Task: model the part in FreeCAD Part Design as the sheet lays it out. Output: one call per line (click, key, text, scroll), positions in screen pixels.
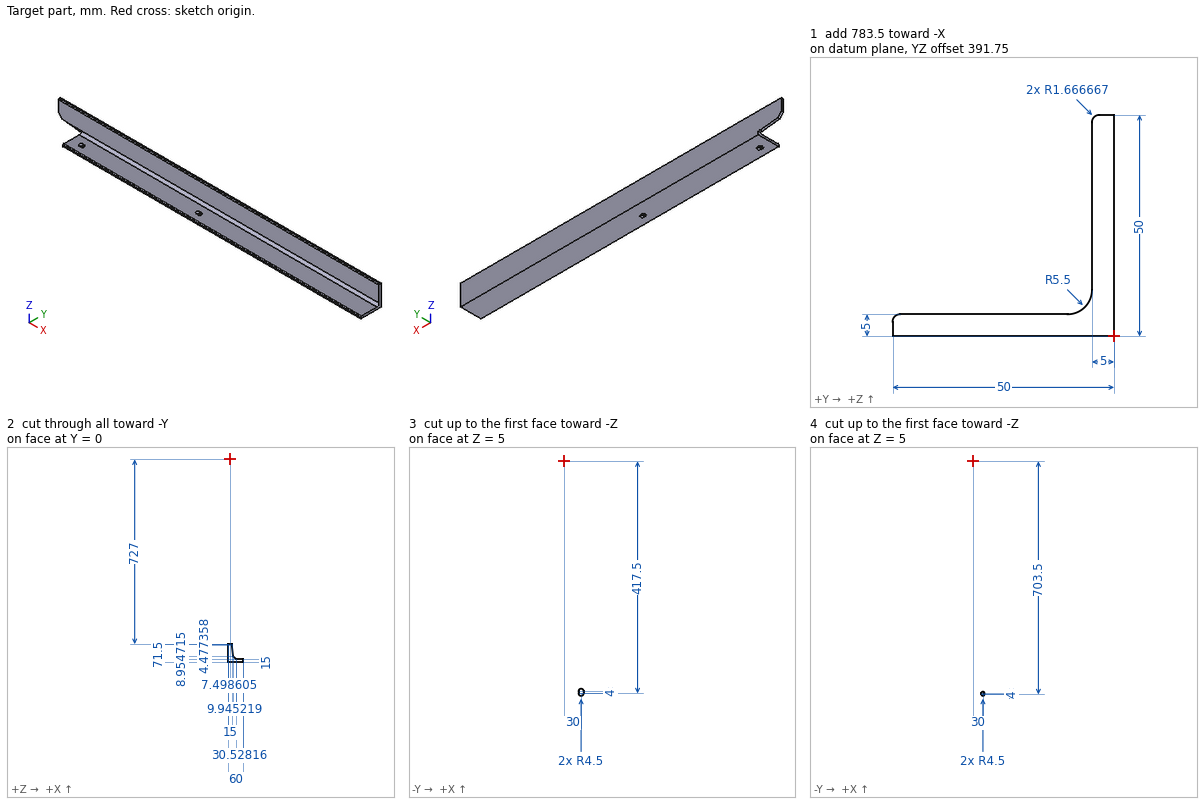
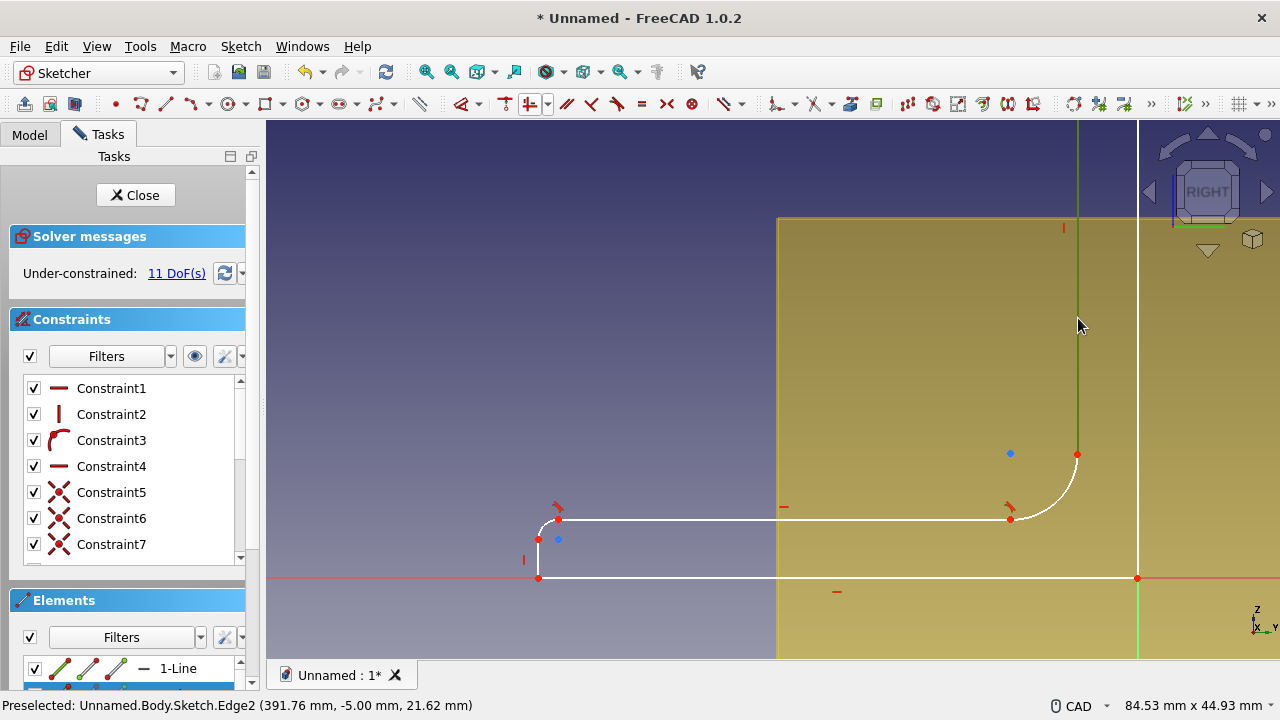
click(1041, 513)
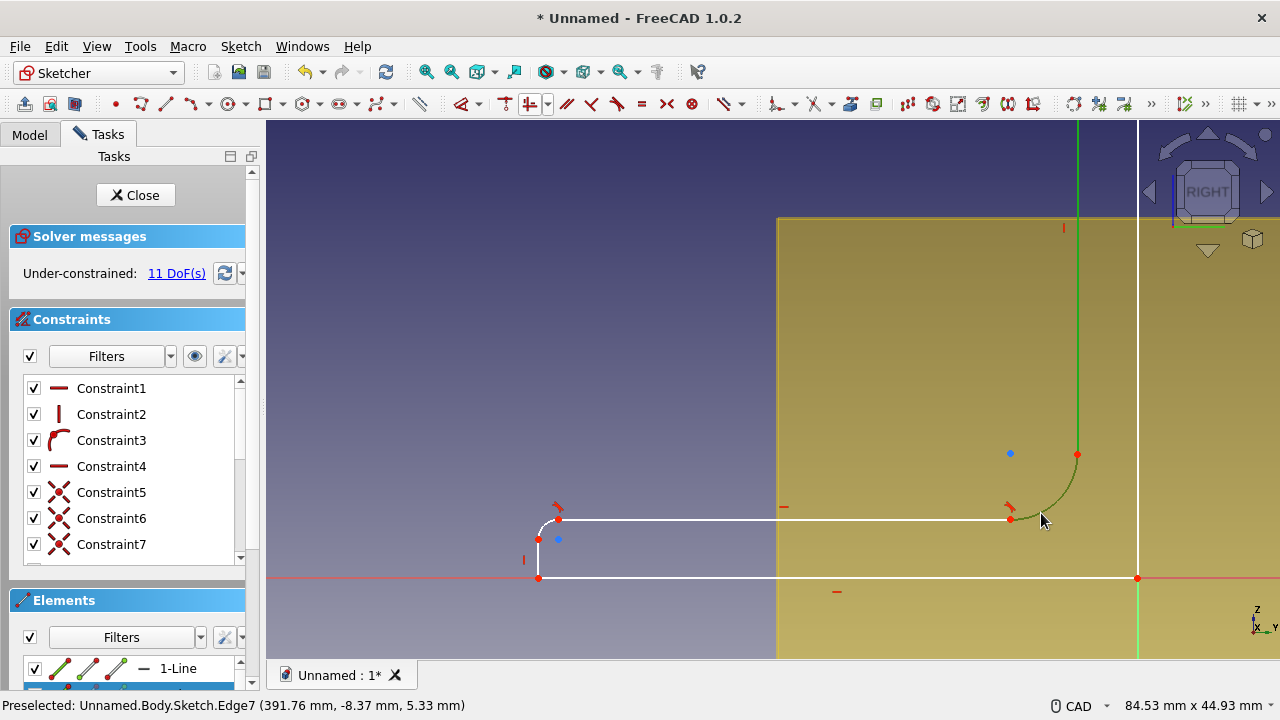
click(617, 104)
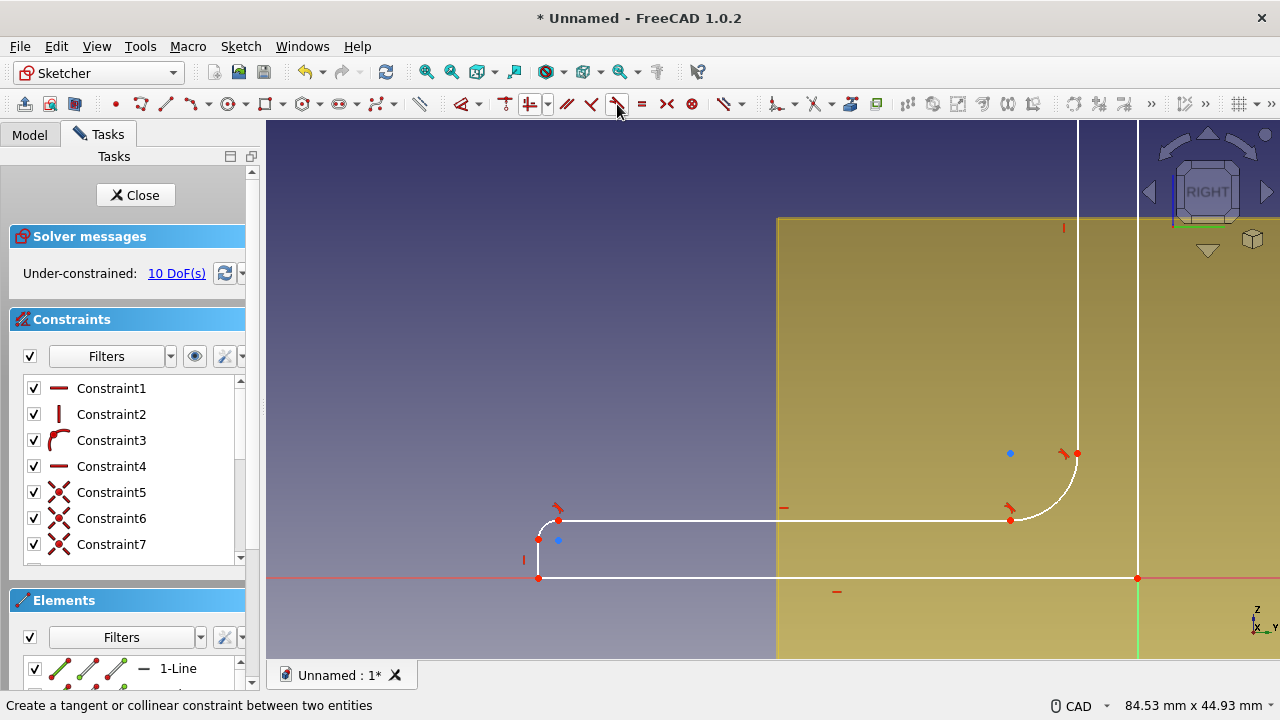
click(1078, 318)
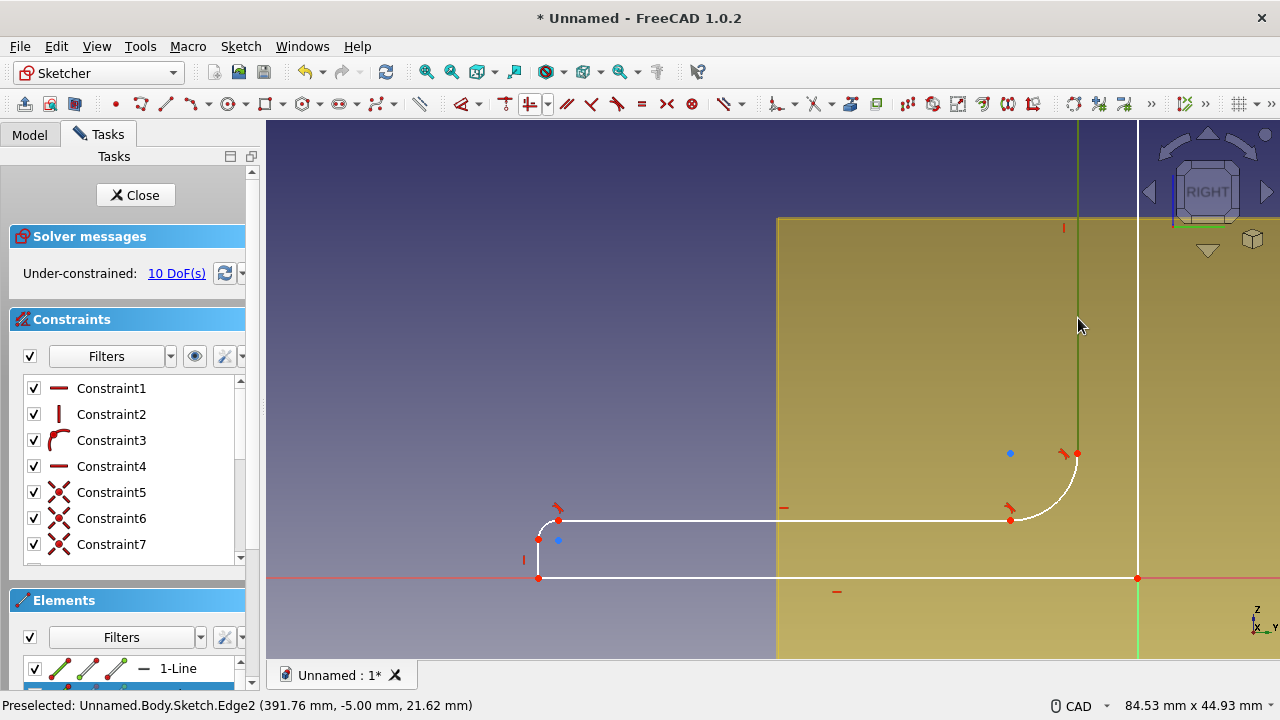
scroll(542, 525, down, 3)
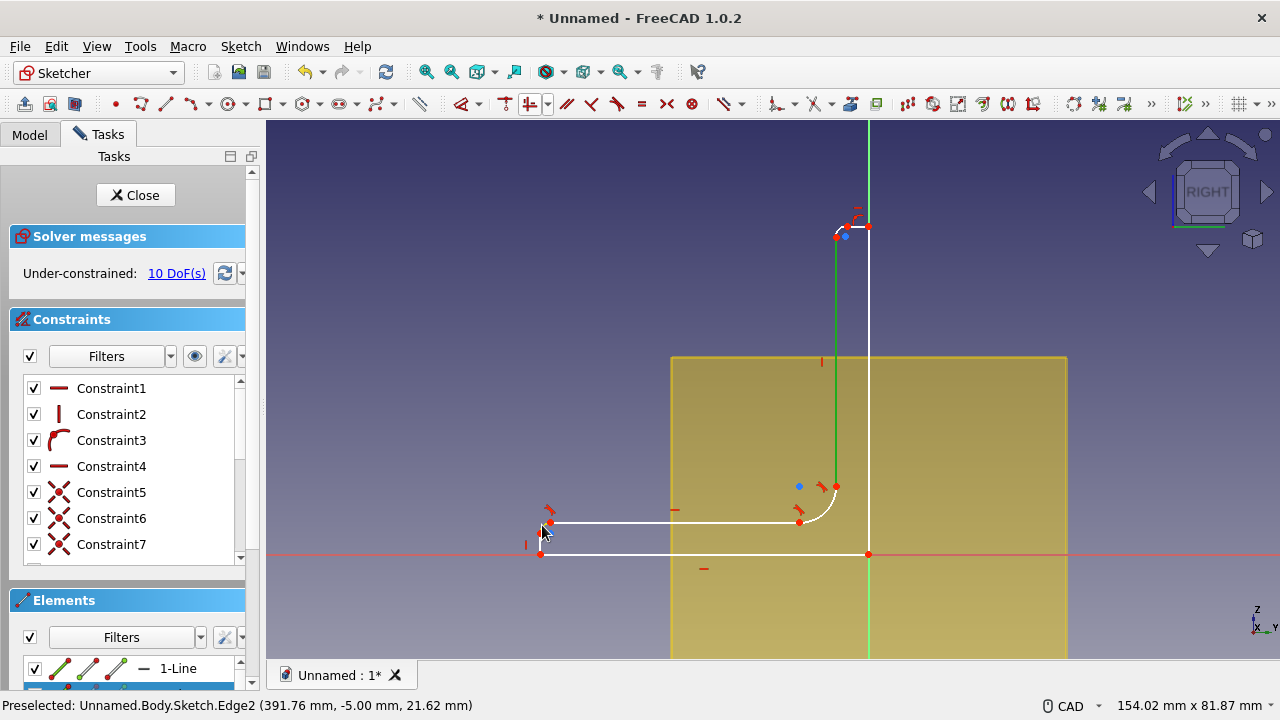
scroll(842, 227, up, 5)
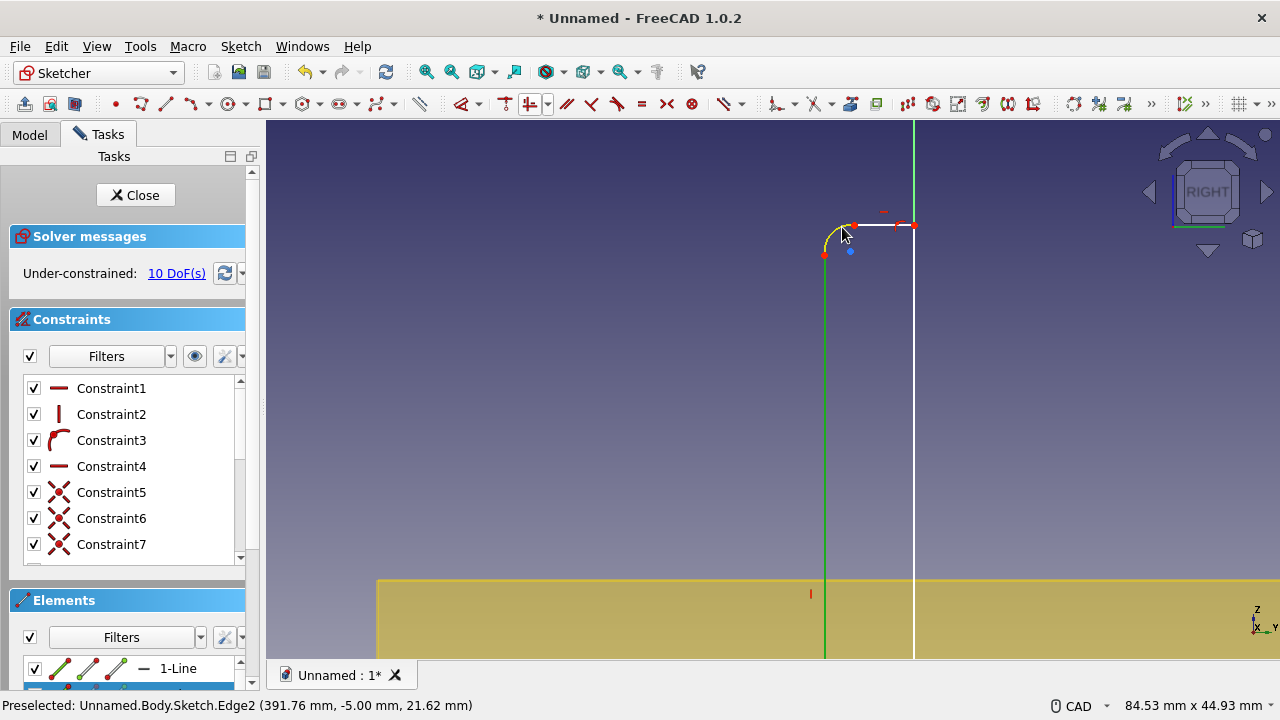
click(840, 227)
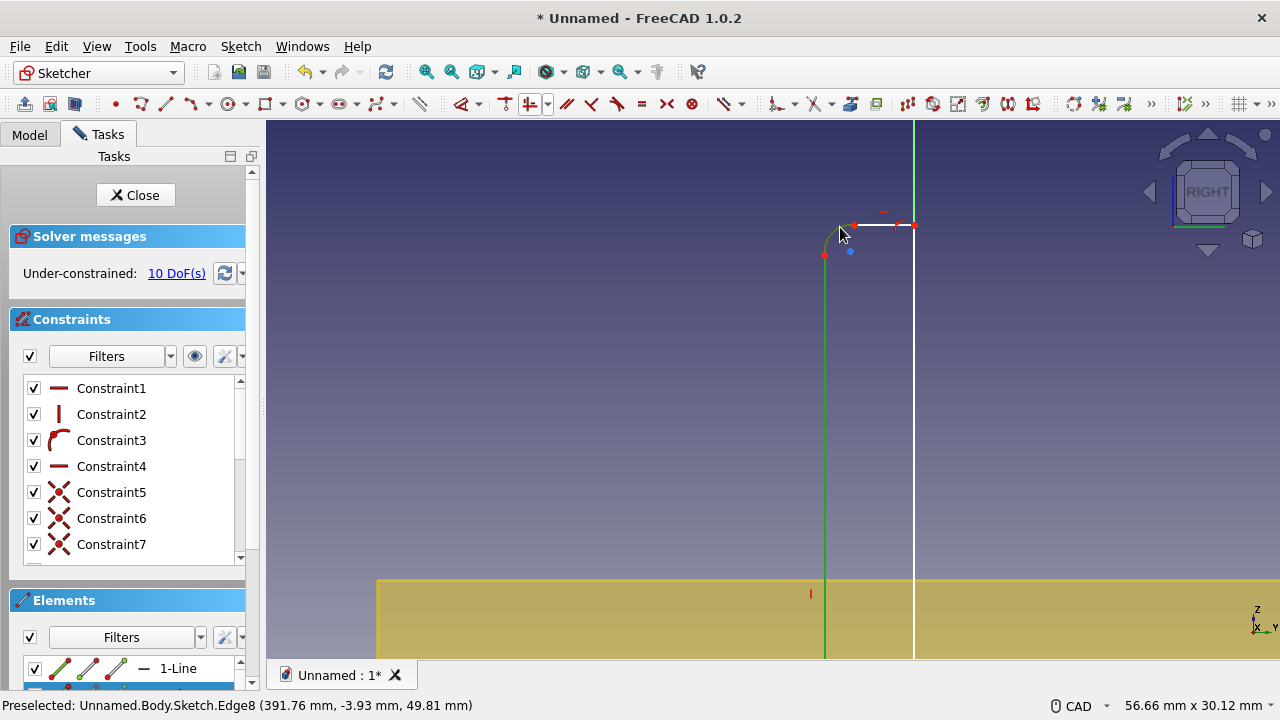
click(617, 104)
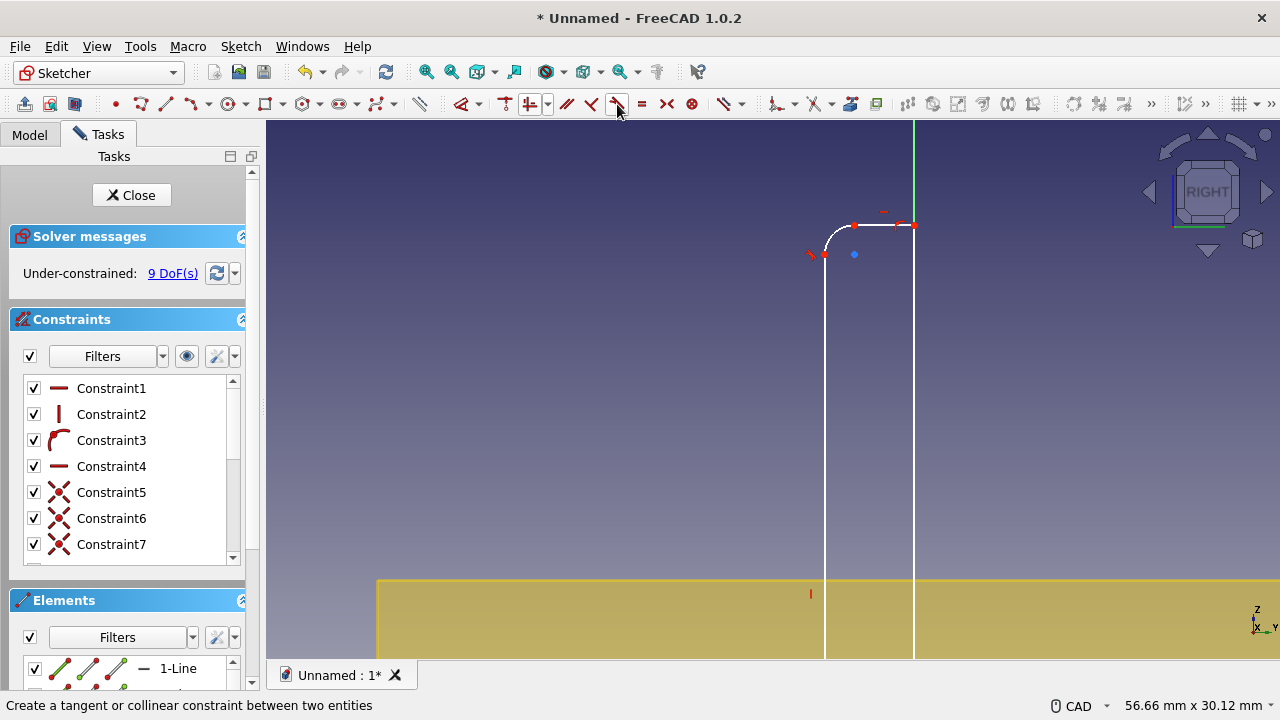
click(873, 225)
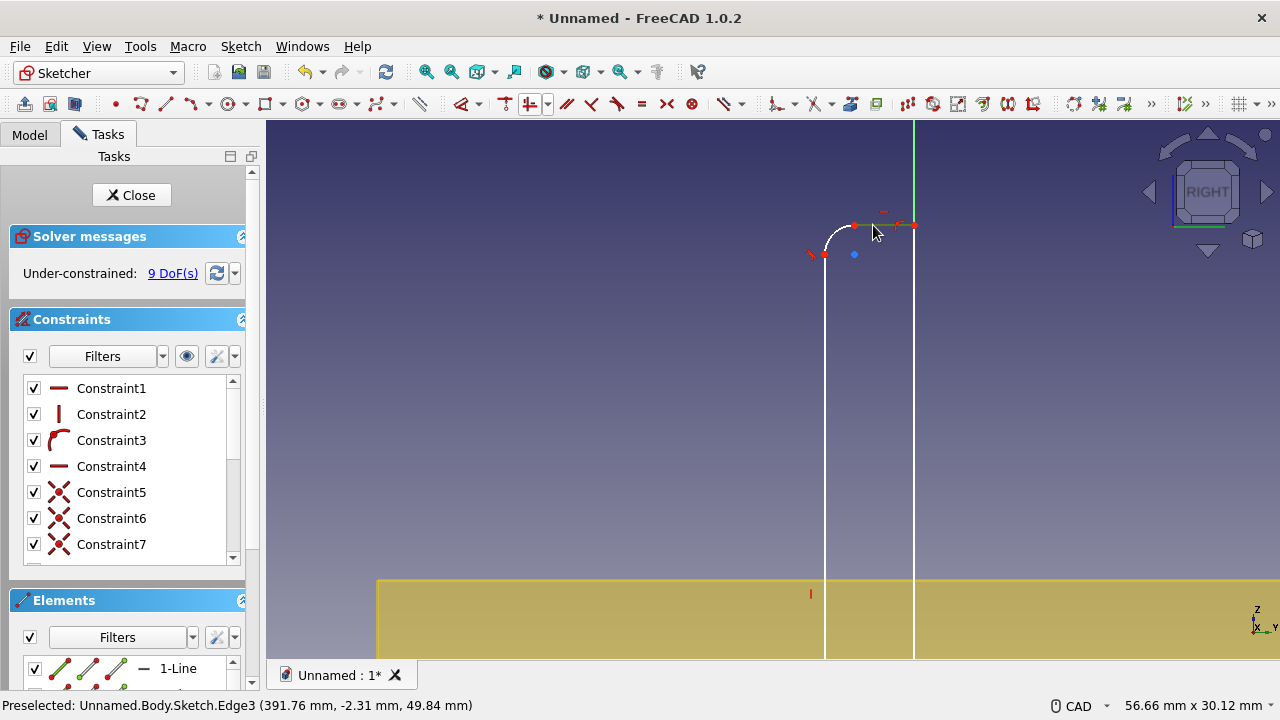
click(841, 228)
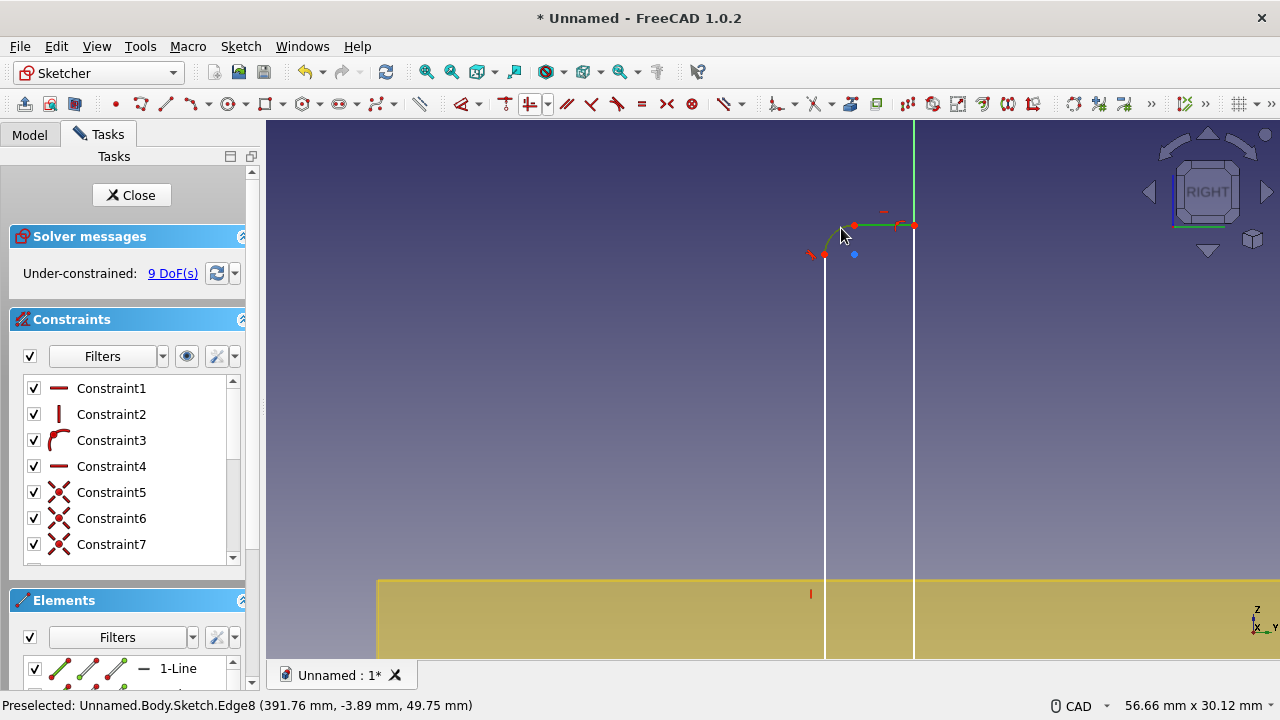
click(617, 104)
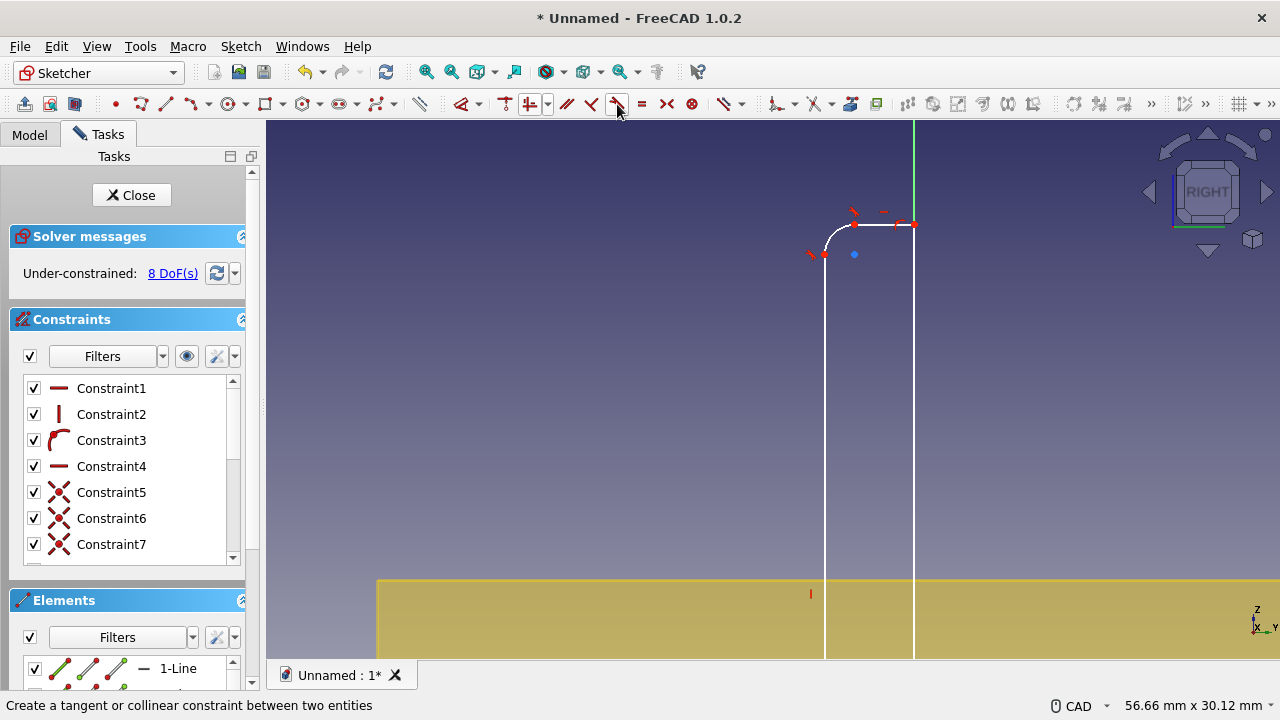
scroll(843, 226, down, 5)